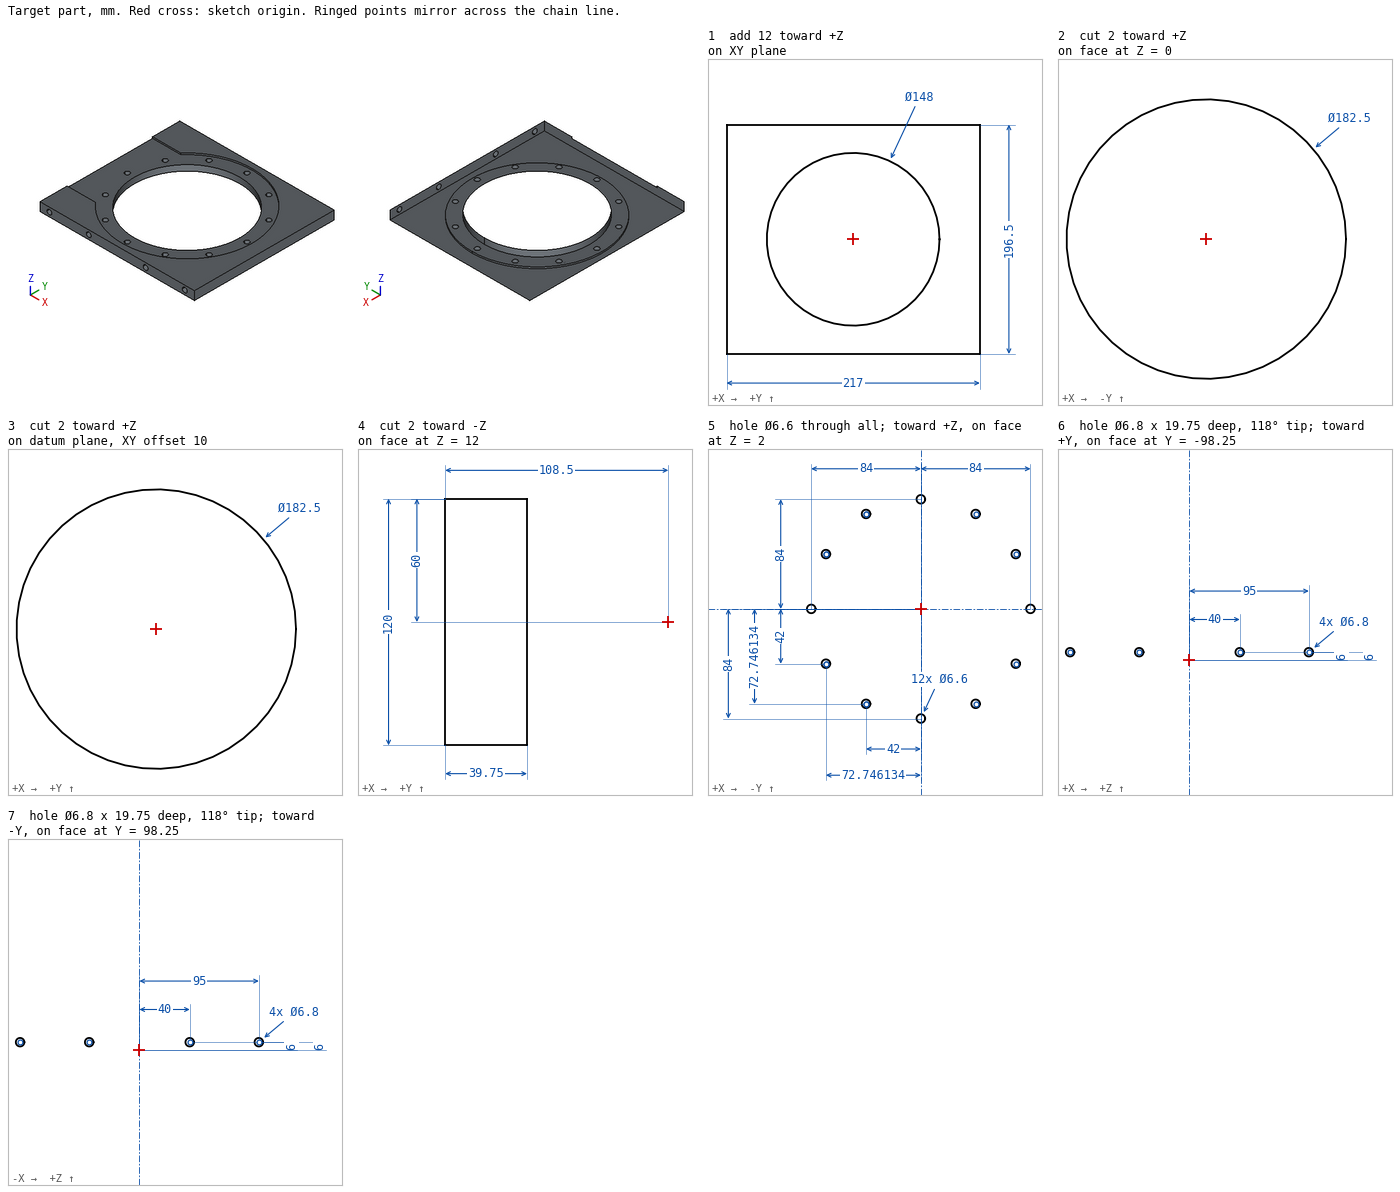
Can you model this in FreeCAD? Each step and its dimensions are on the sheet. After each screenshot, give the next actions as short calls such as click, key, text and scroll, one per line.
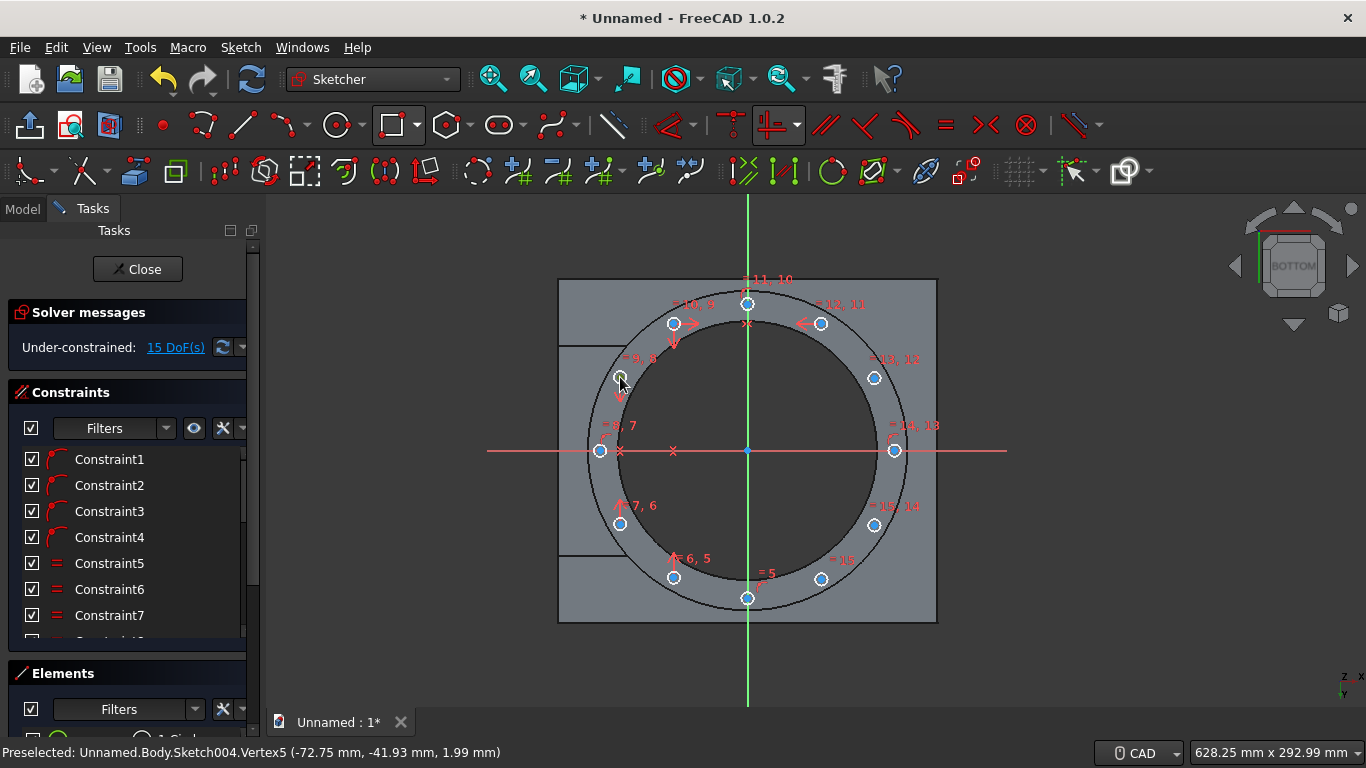
click(874, 378)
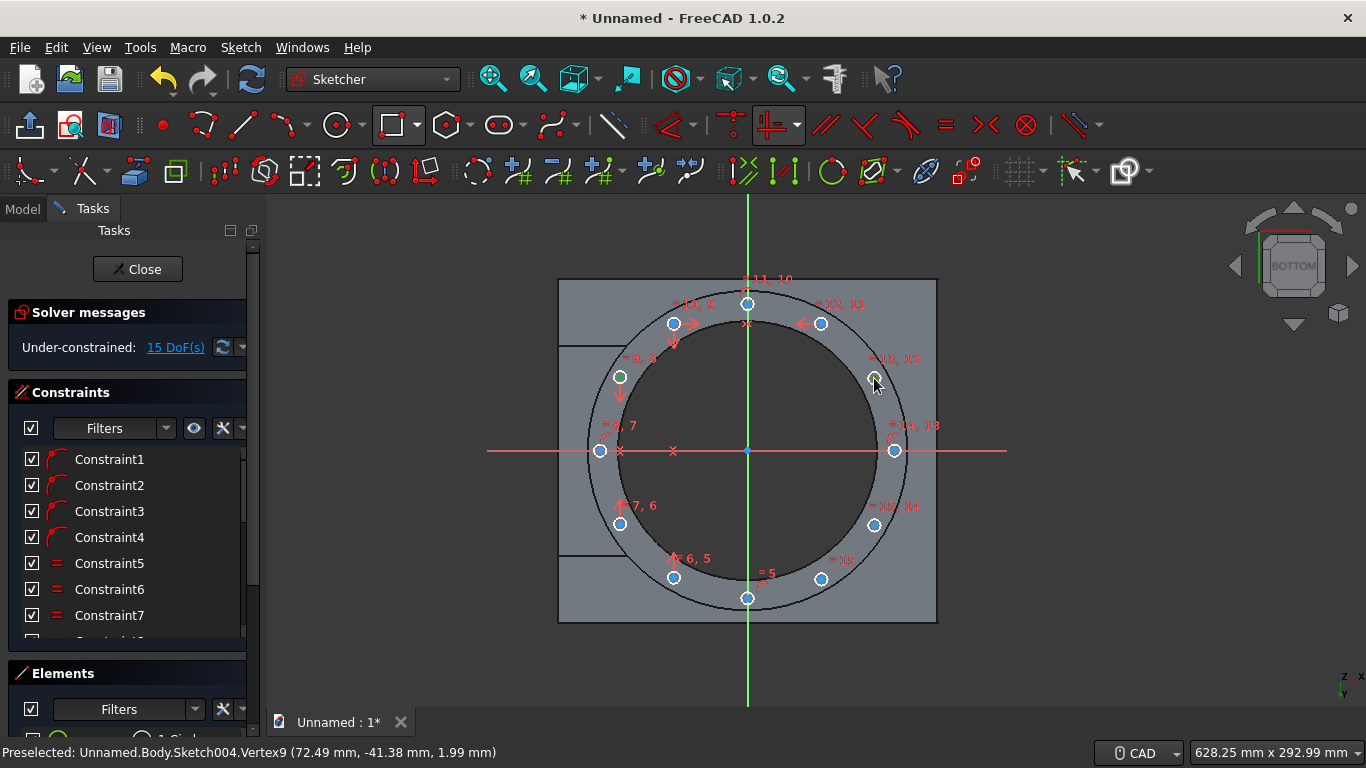
click(748, 646)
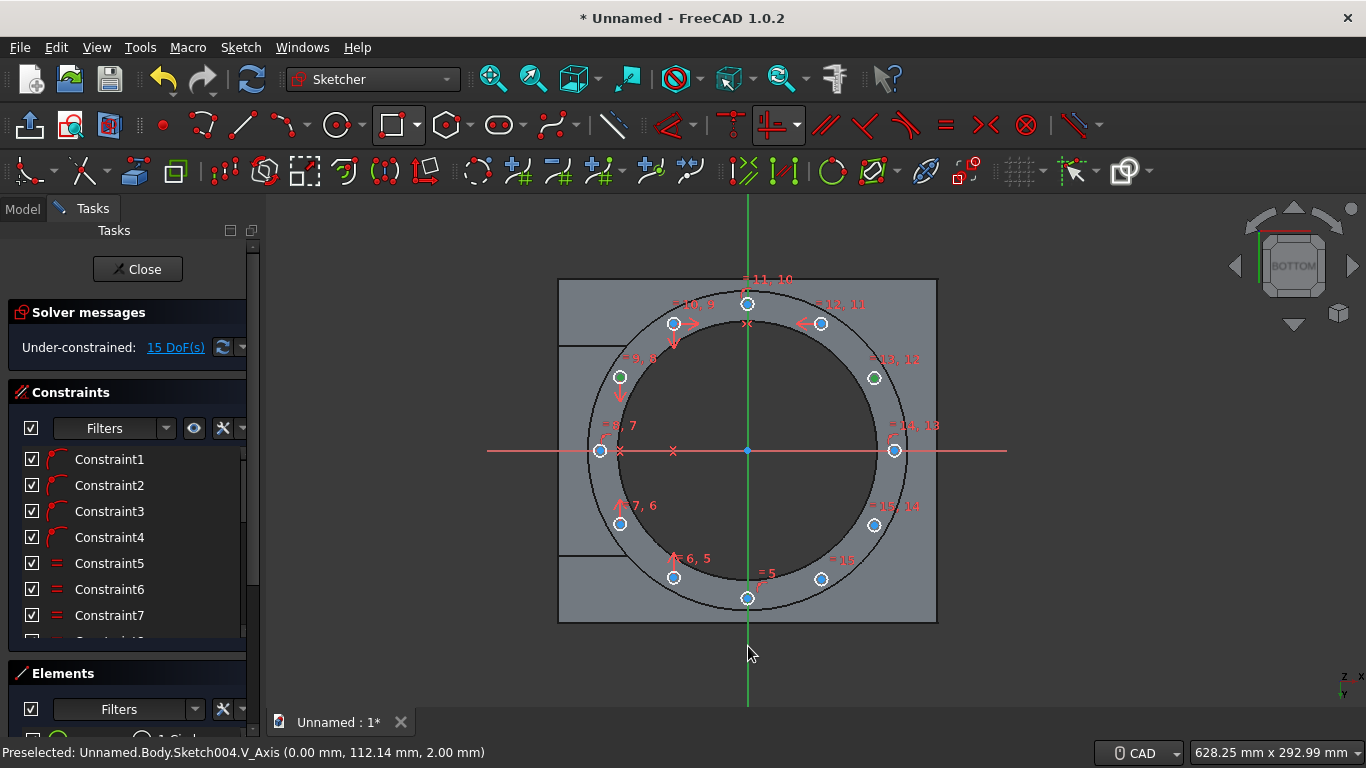
click(986, 126)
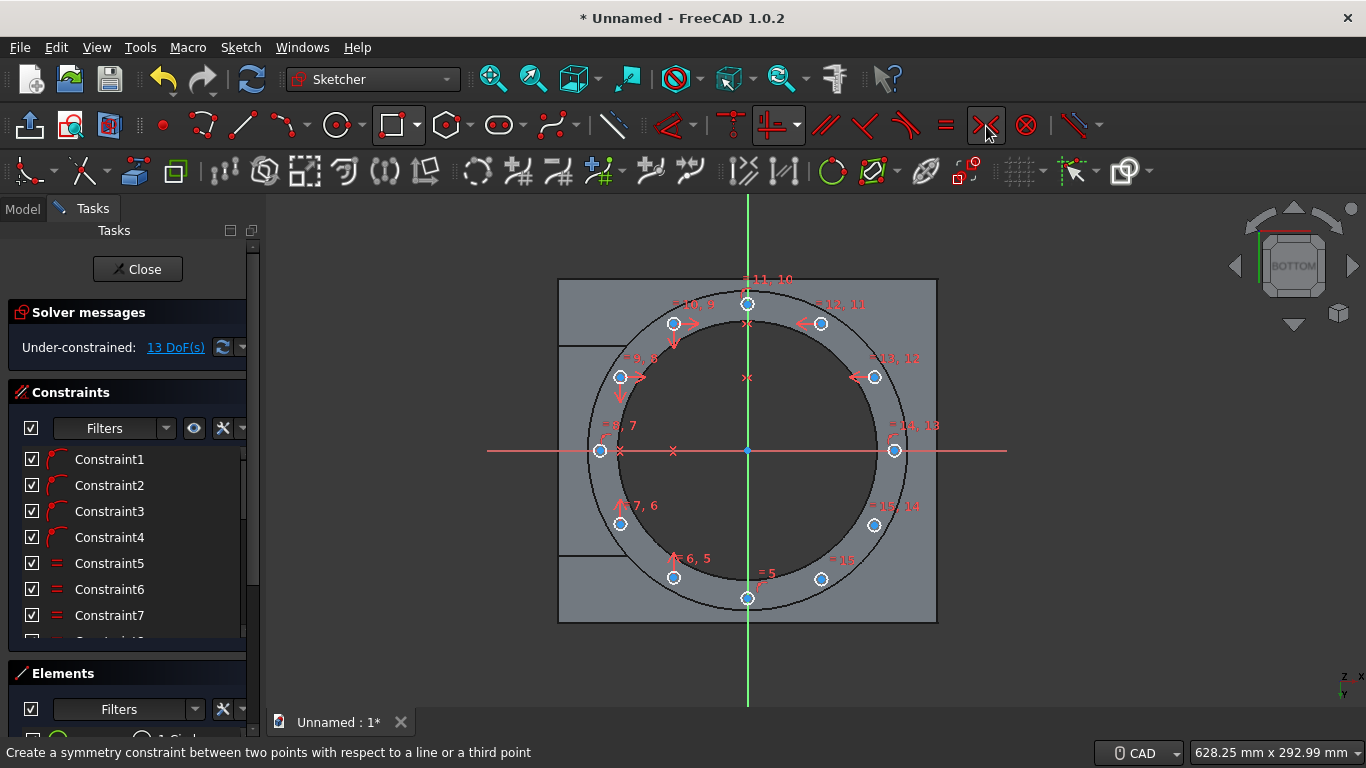
click(620, 524)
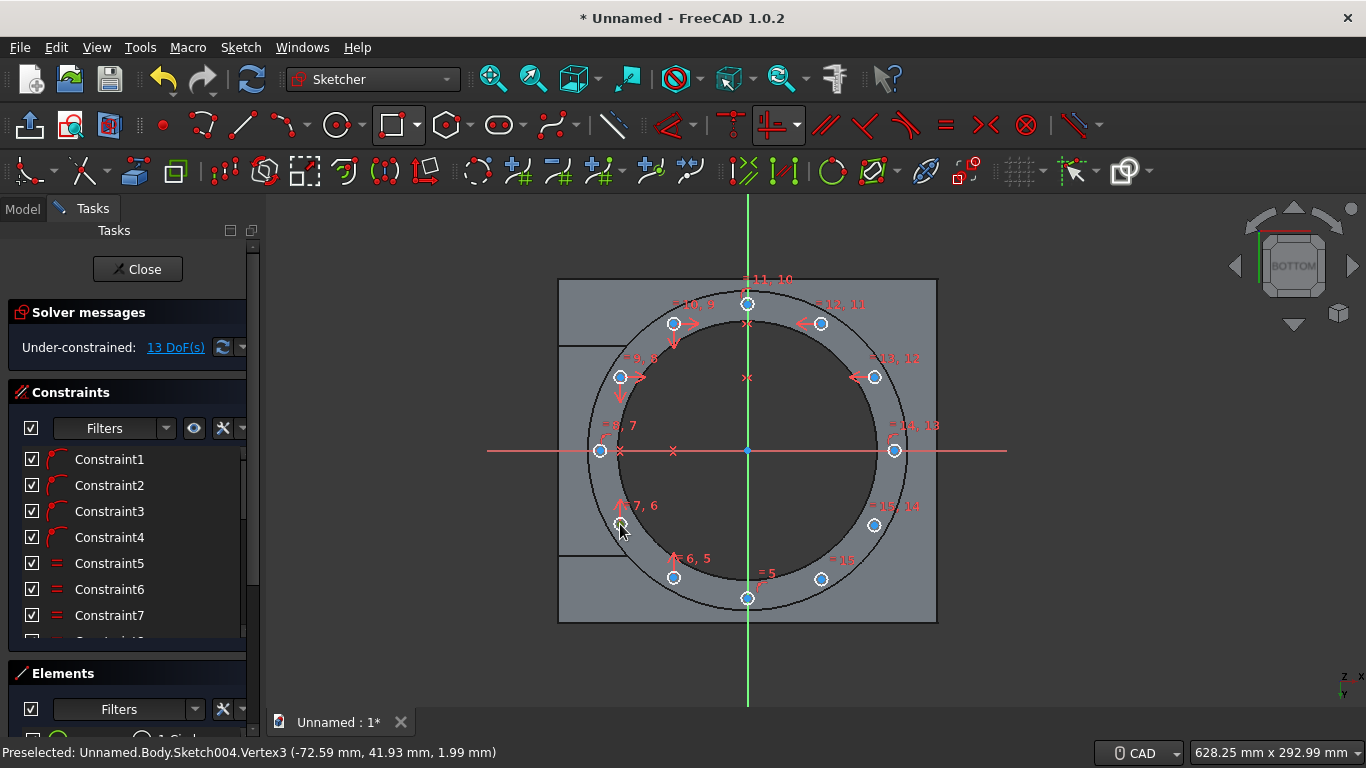
click(874, 525)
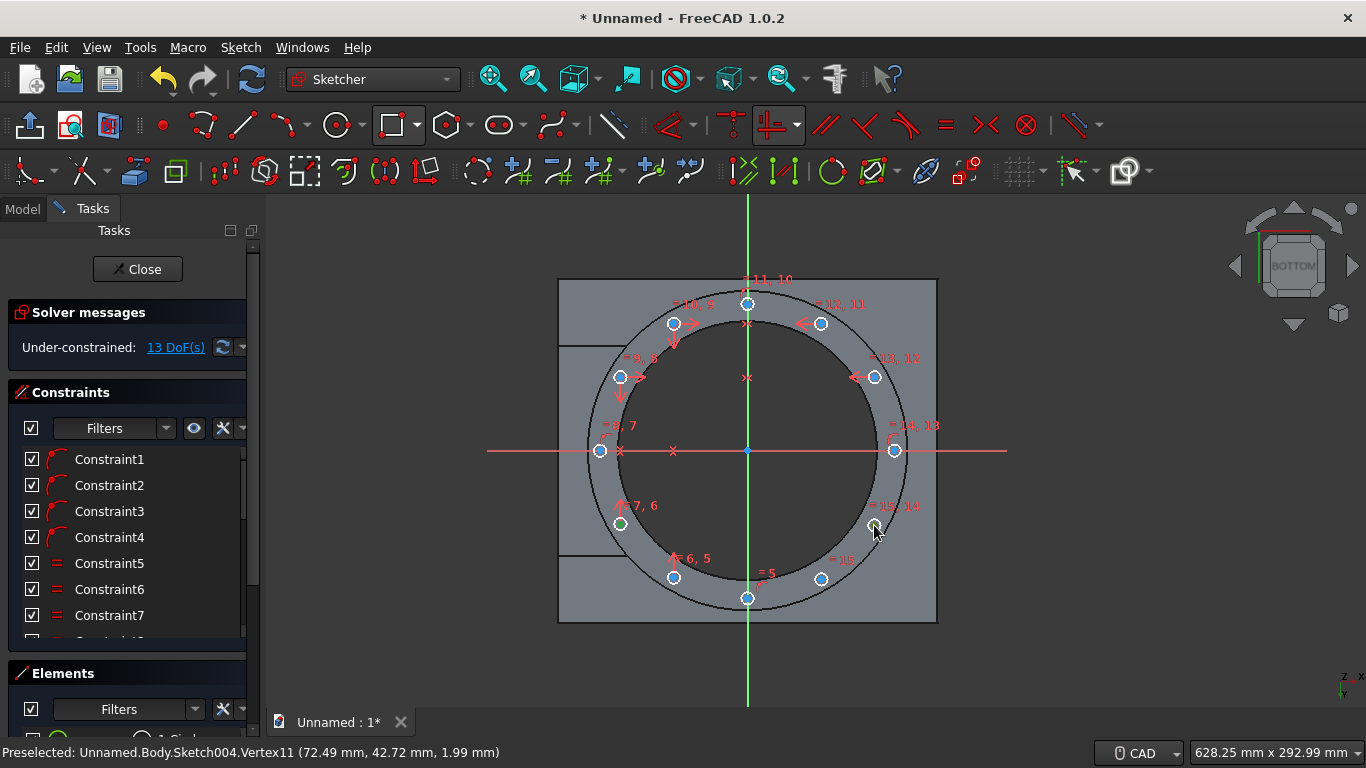
click(748, 646)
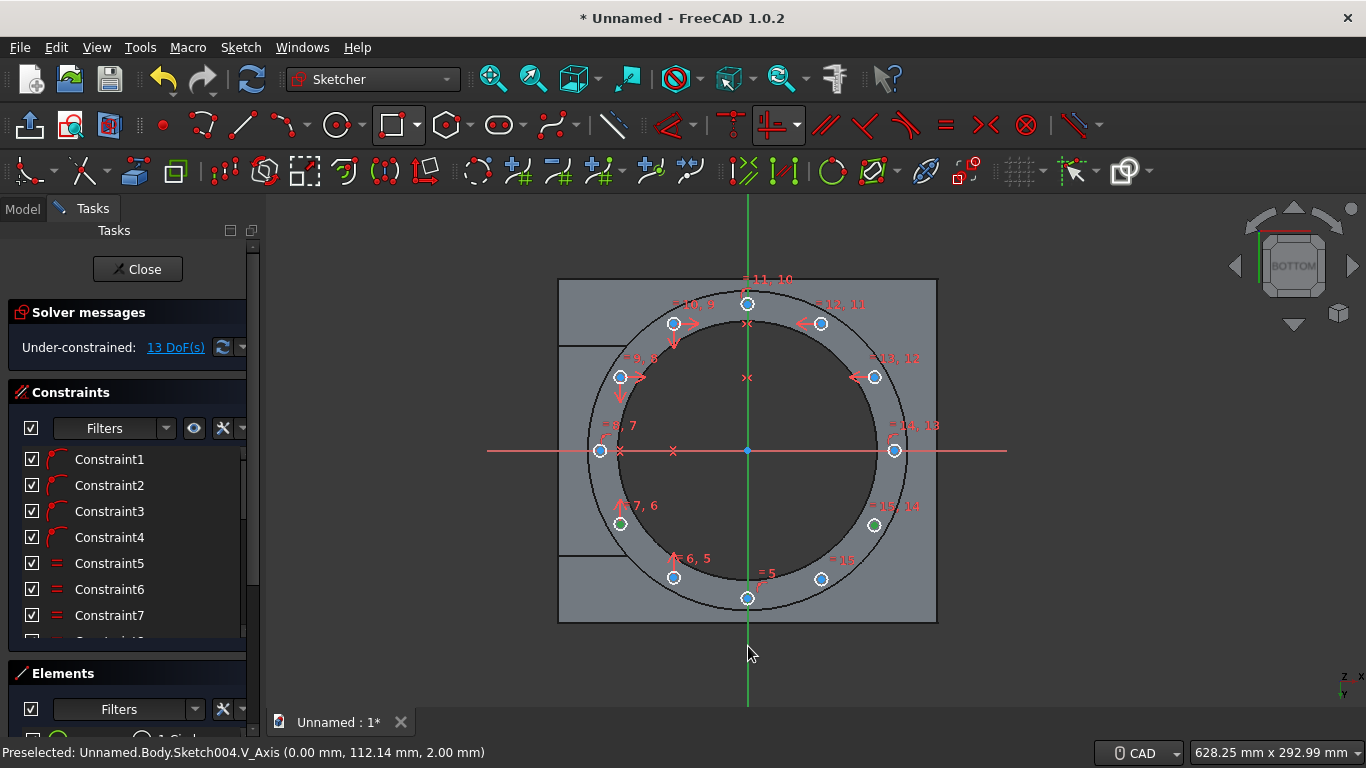
click(986, 126)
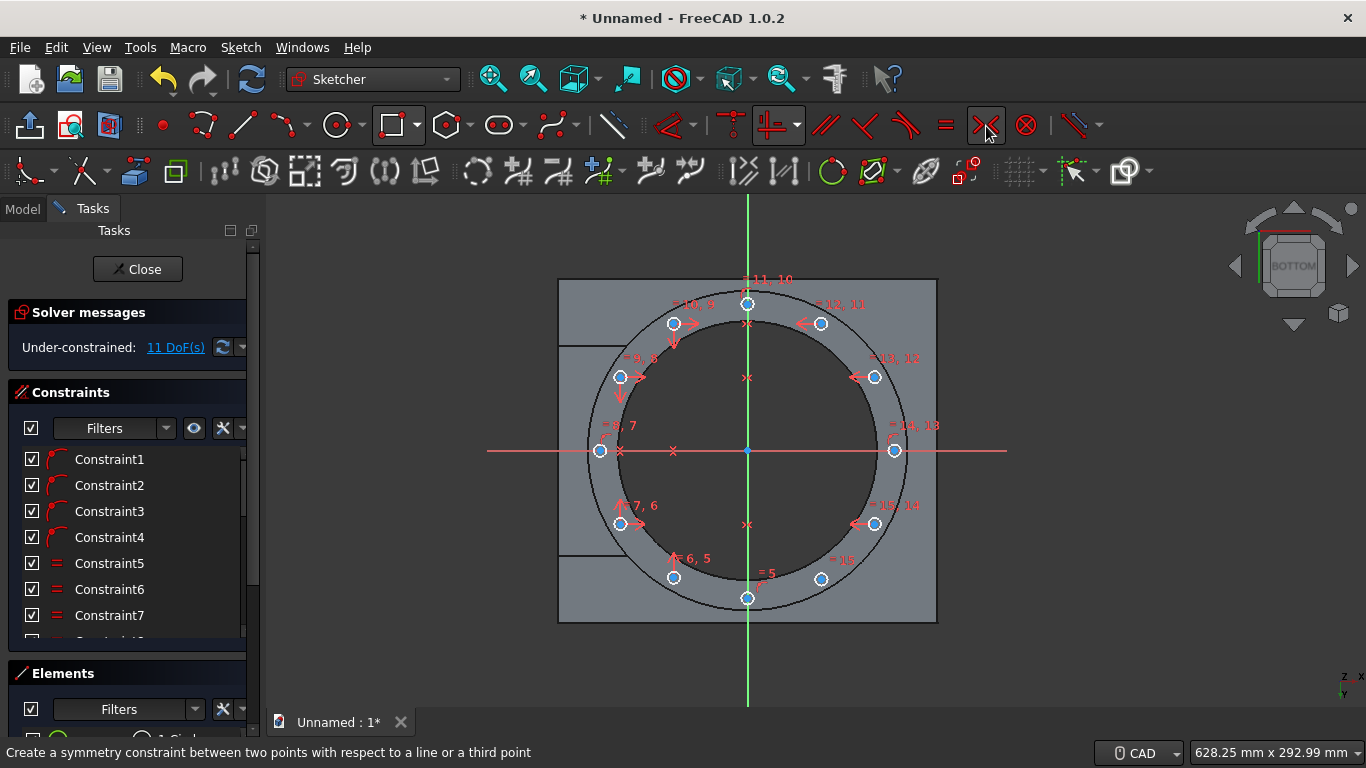
click(674, 578)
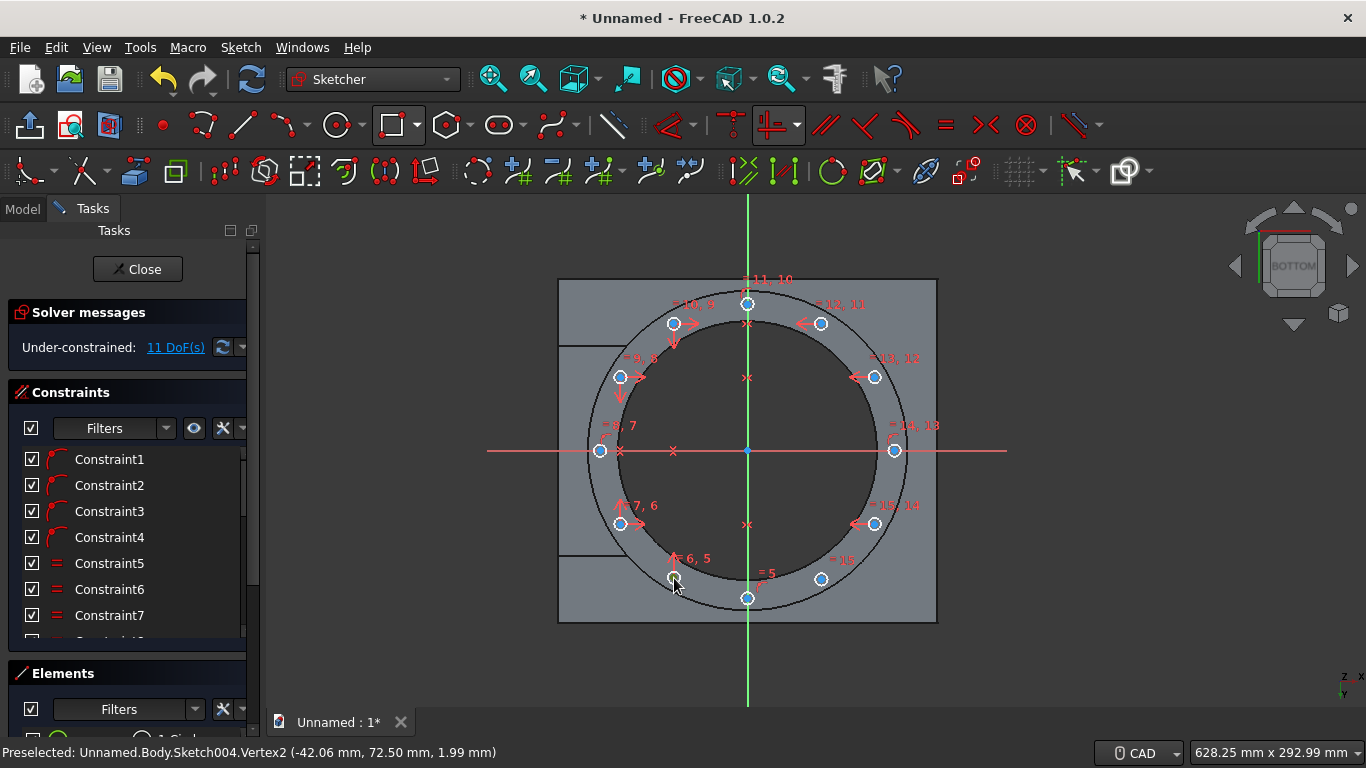
click(821, 579)